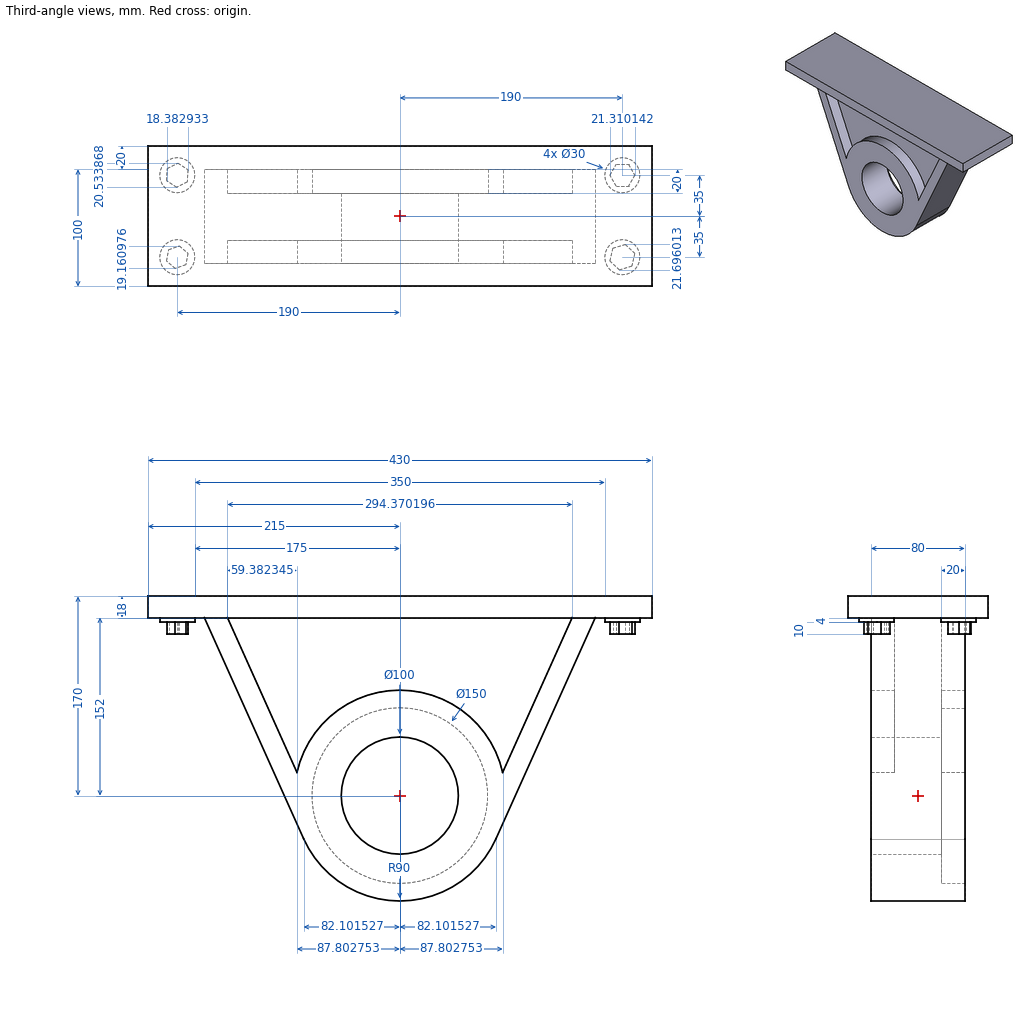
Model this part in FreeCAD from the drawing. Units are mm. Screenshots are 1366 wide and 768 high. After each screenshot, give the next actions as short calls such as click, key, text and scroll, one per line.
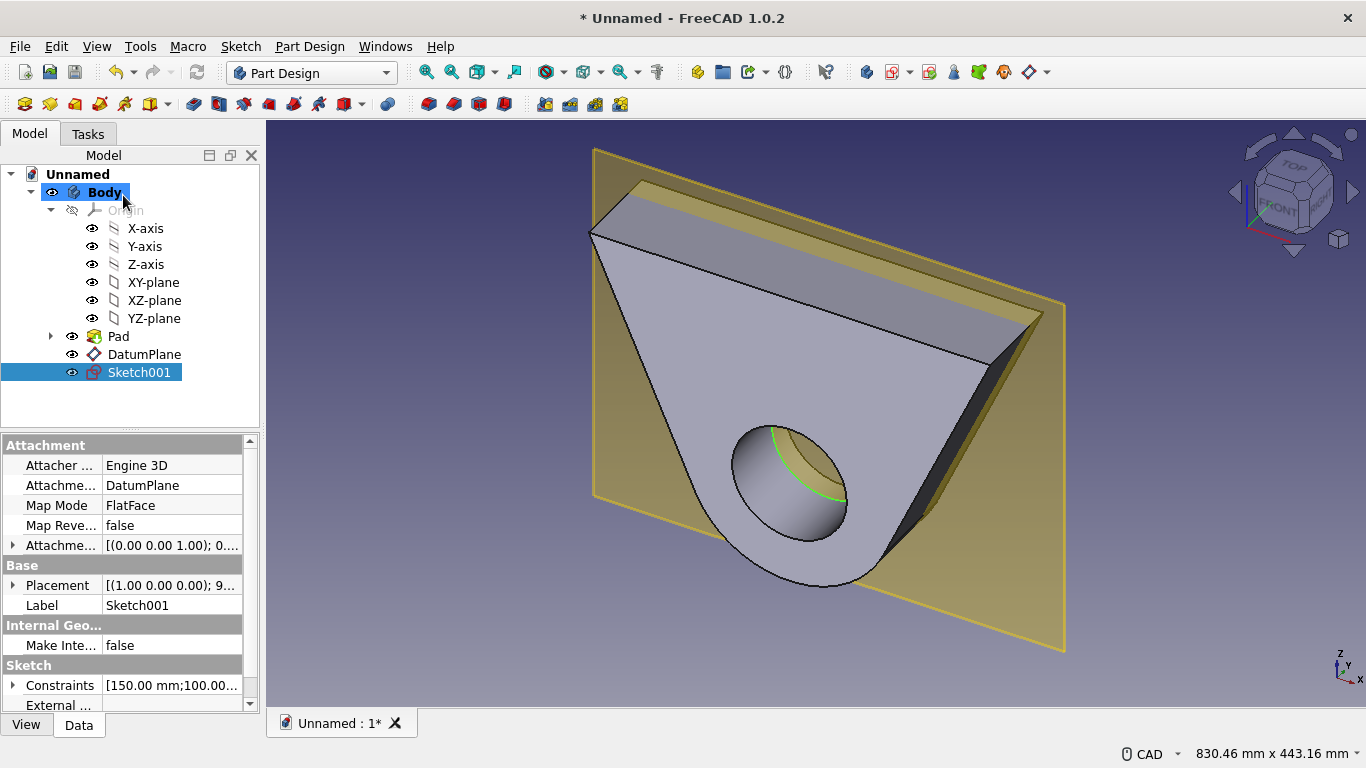
click(194, 104)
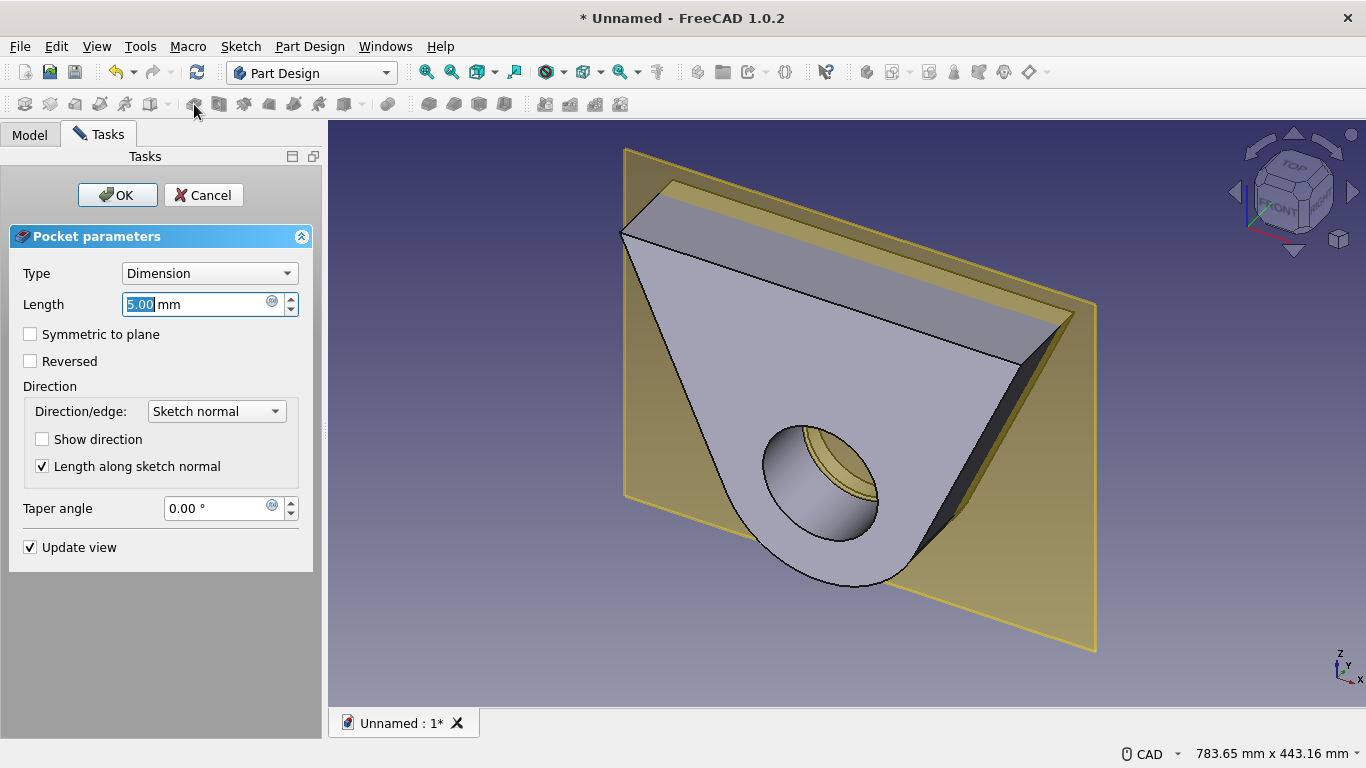
text(20)
key(Tab)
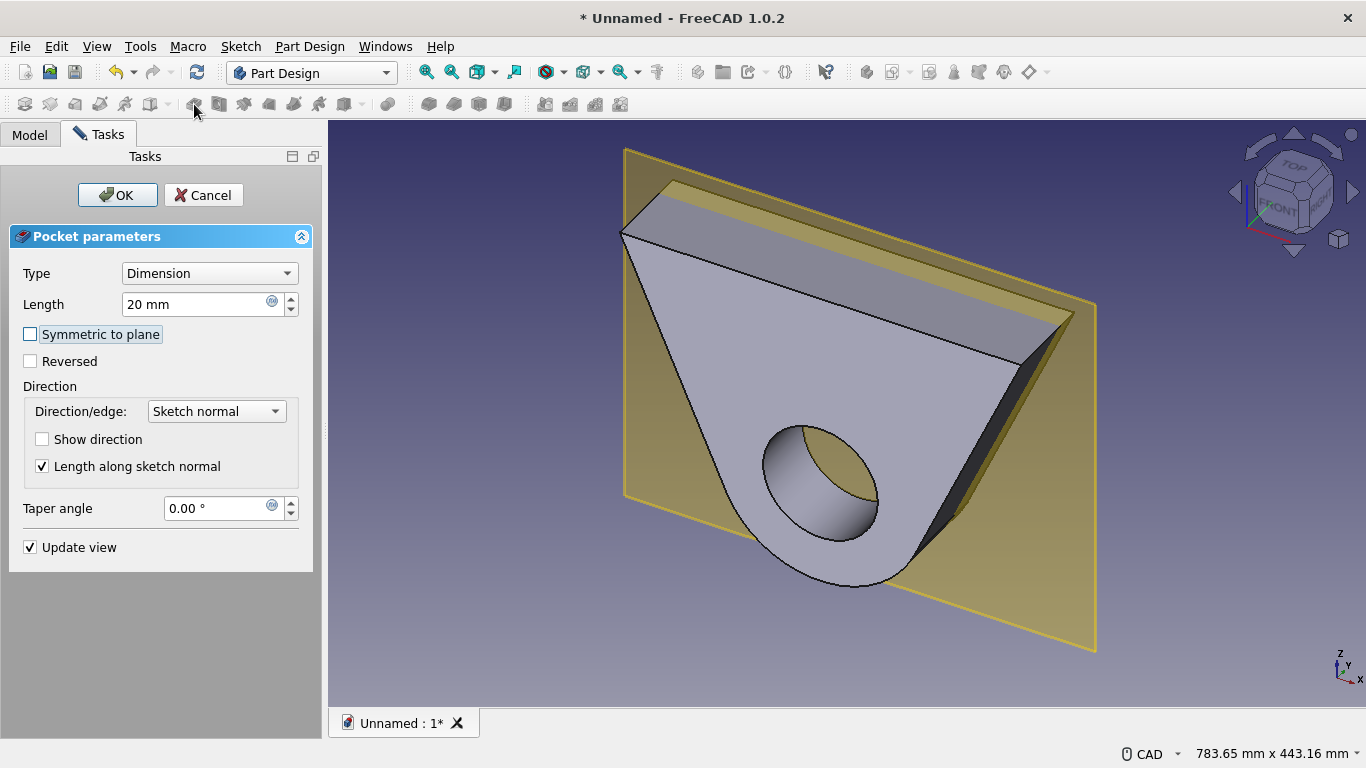
click(118, 195)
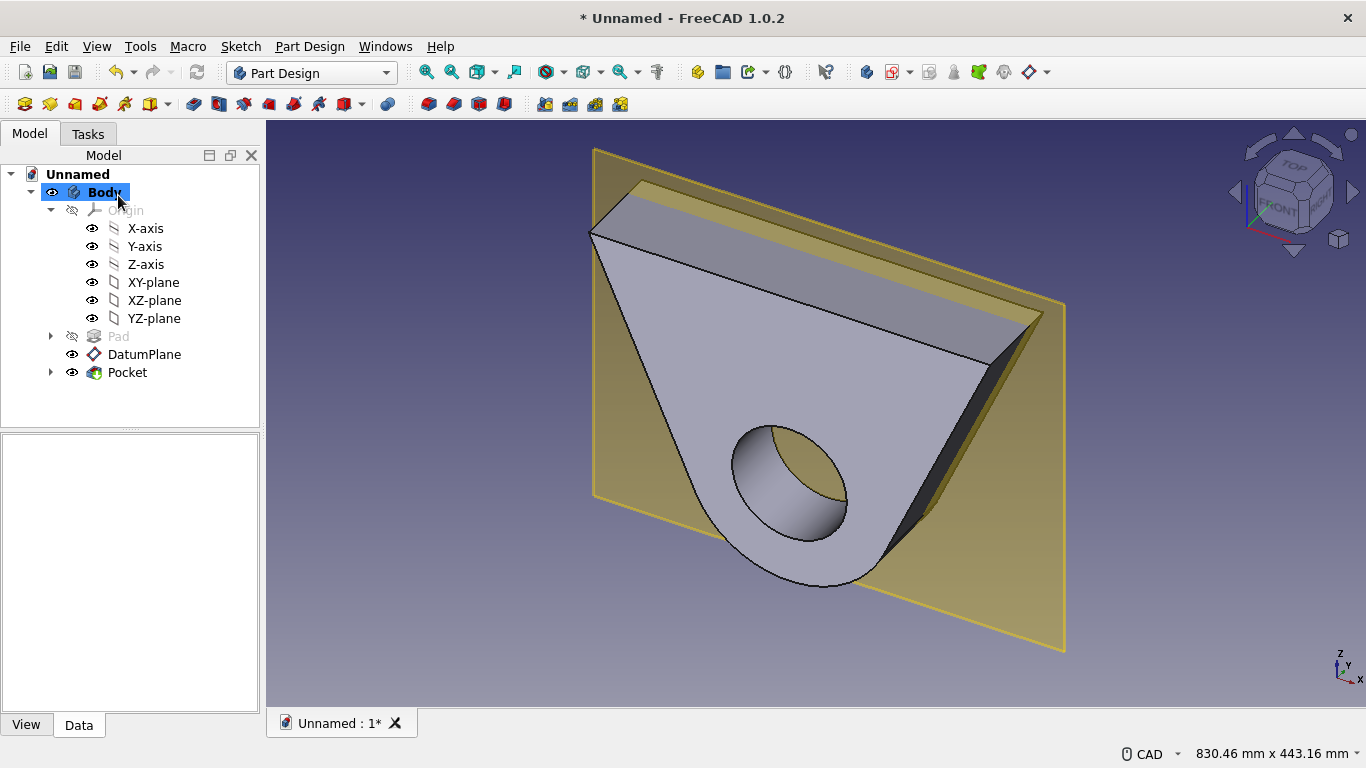
click(117, 354)
key(space)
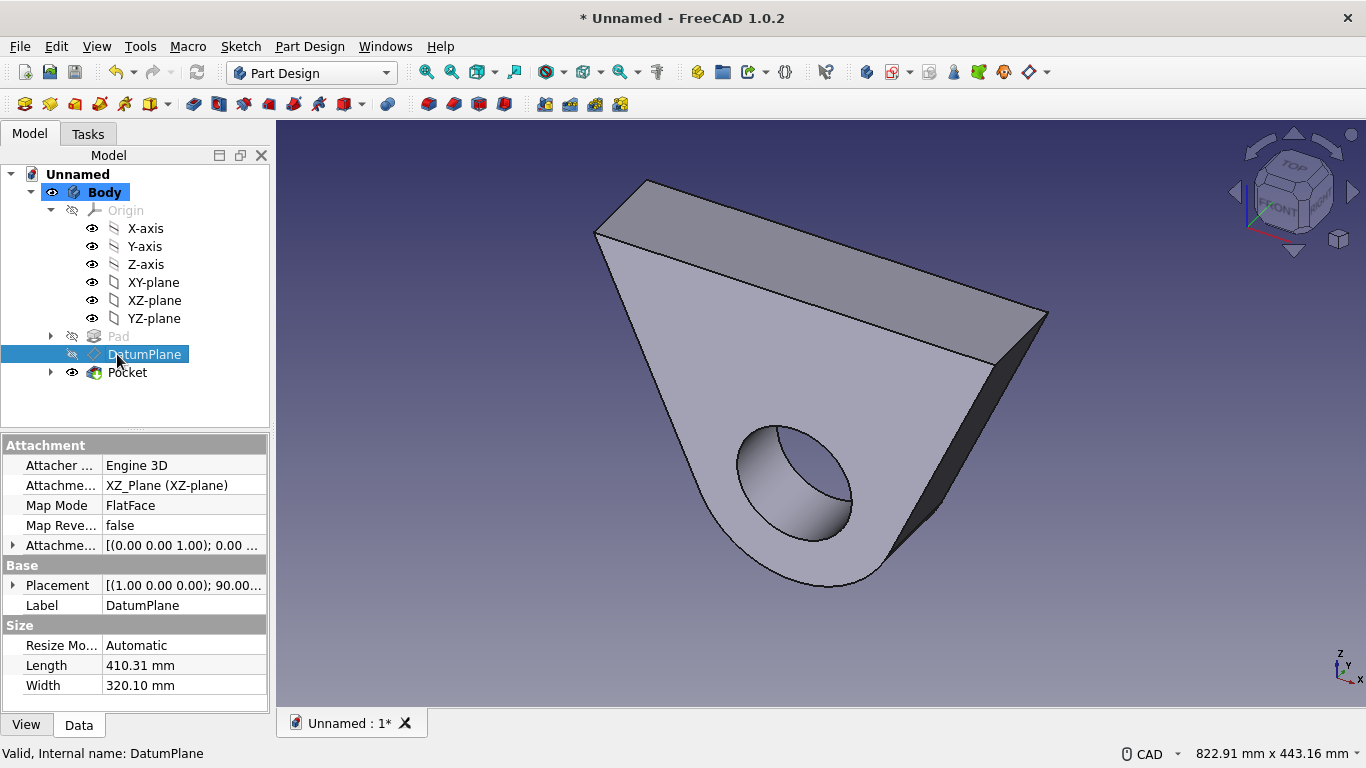
key(4)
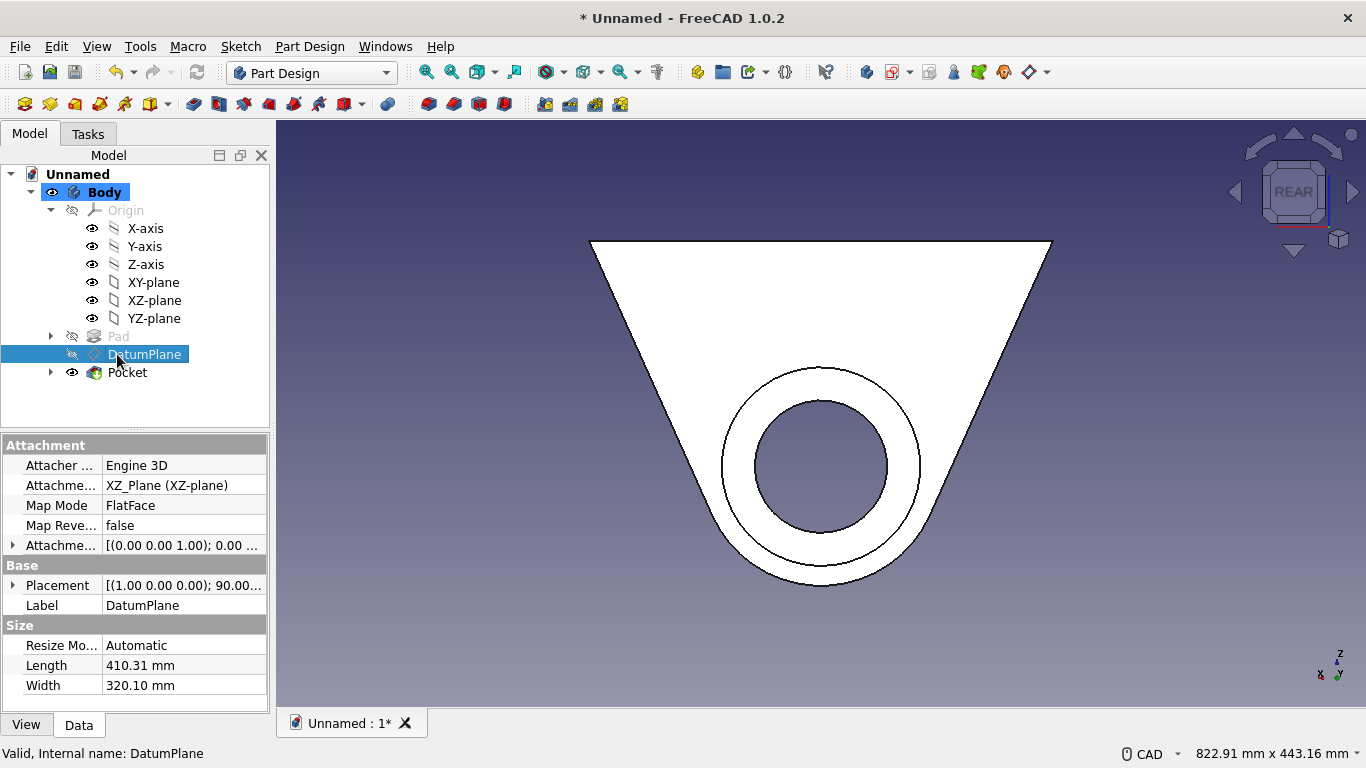
click(736, 466)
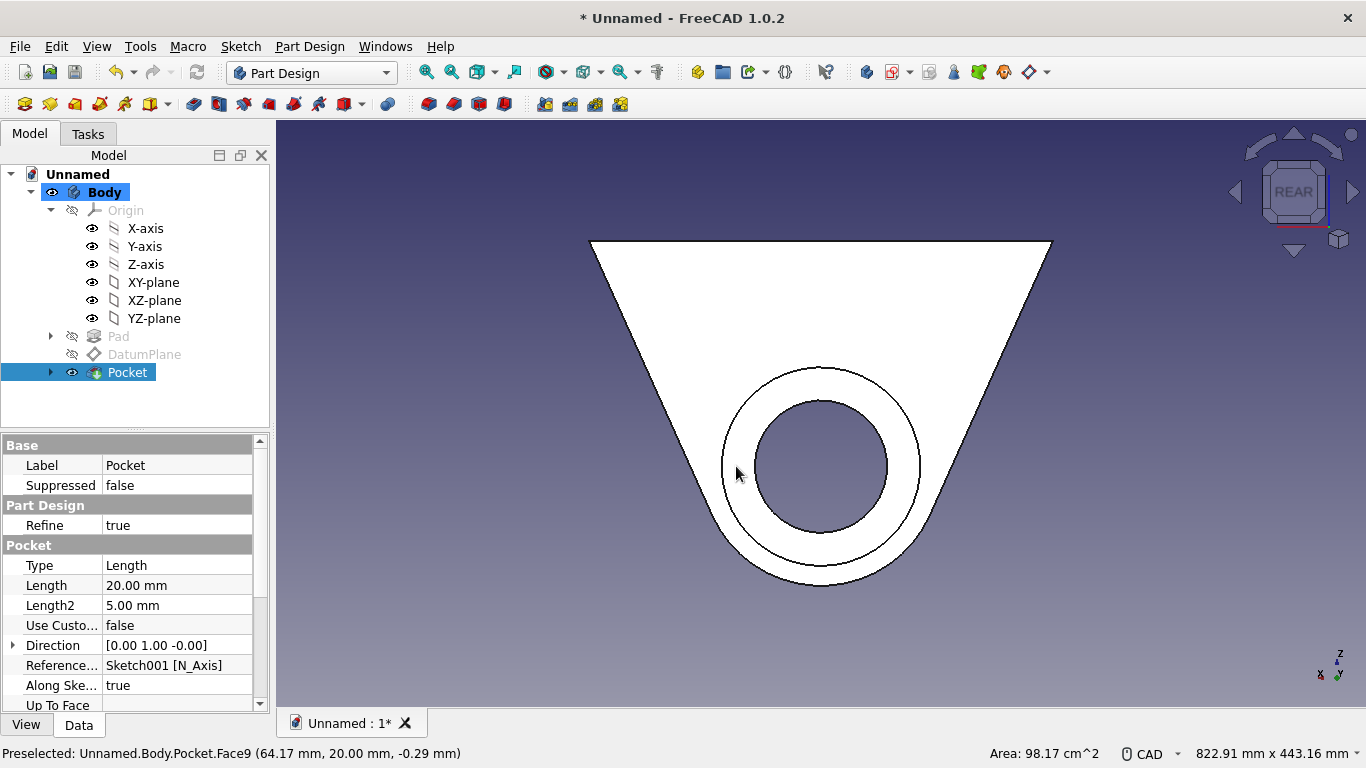
click(892, 72)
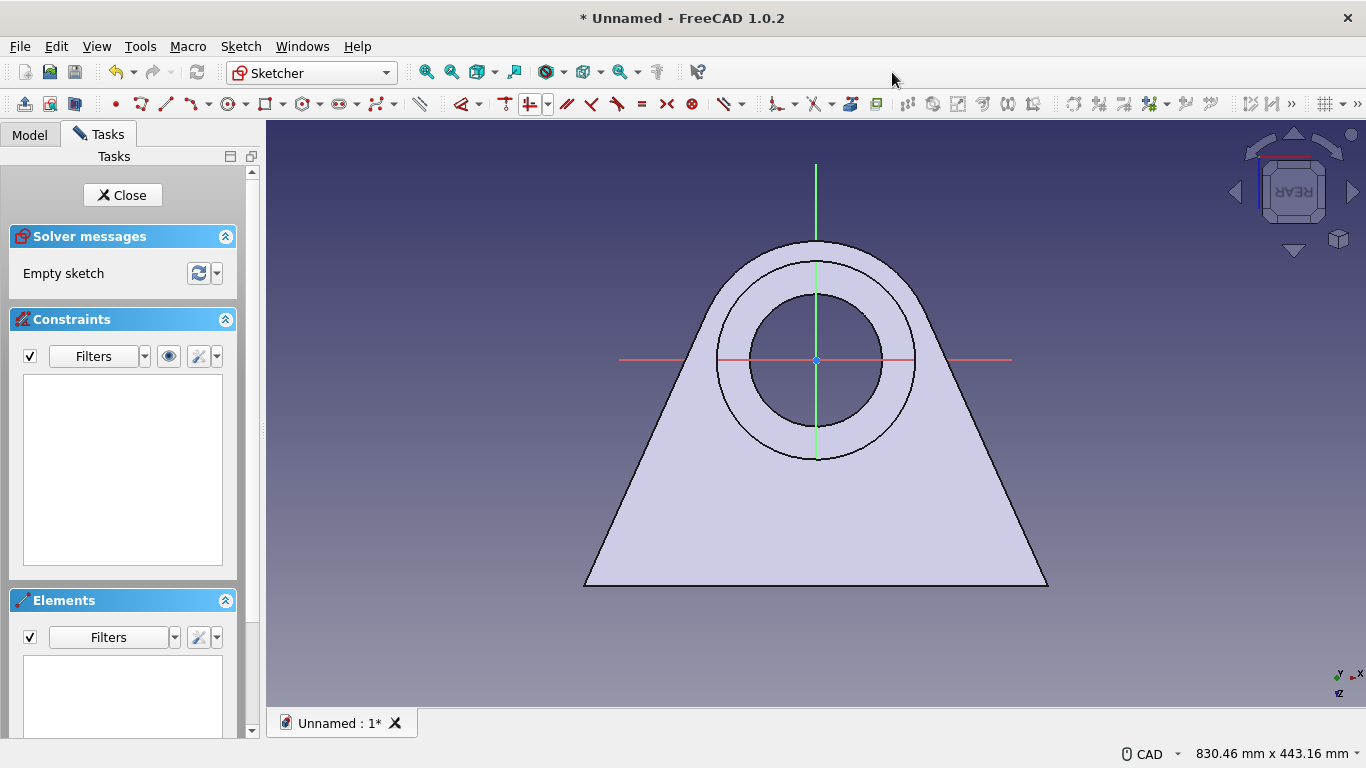
click(75, 104)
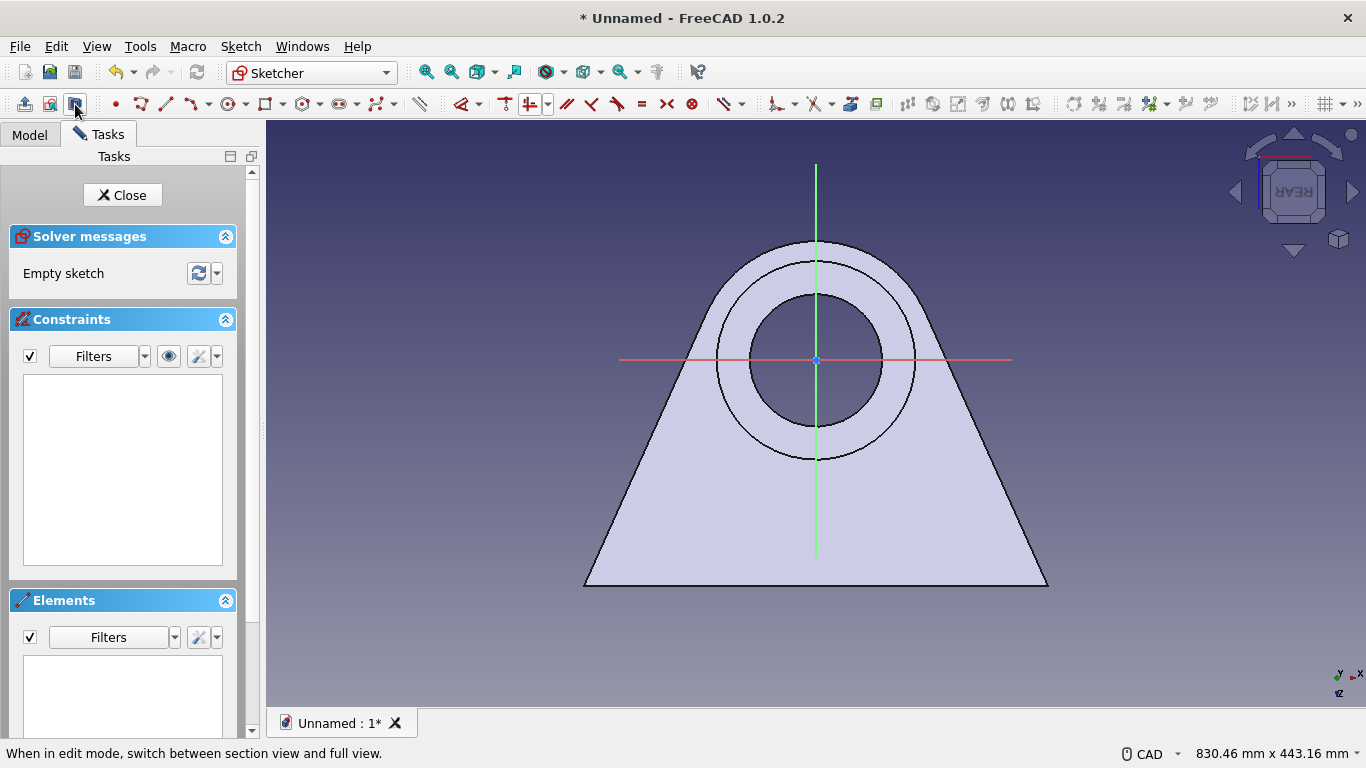
scroll(955, 558, up, 2)